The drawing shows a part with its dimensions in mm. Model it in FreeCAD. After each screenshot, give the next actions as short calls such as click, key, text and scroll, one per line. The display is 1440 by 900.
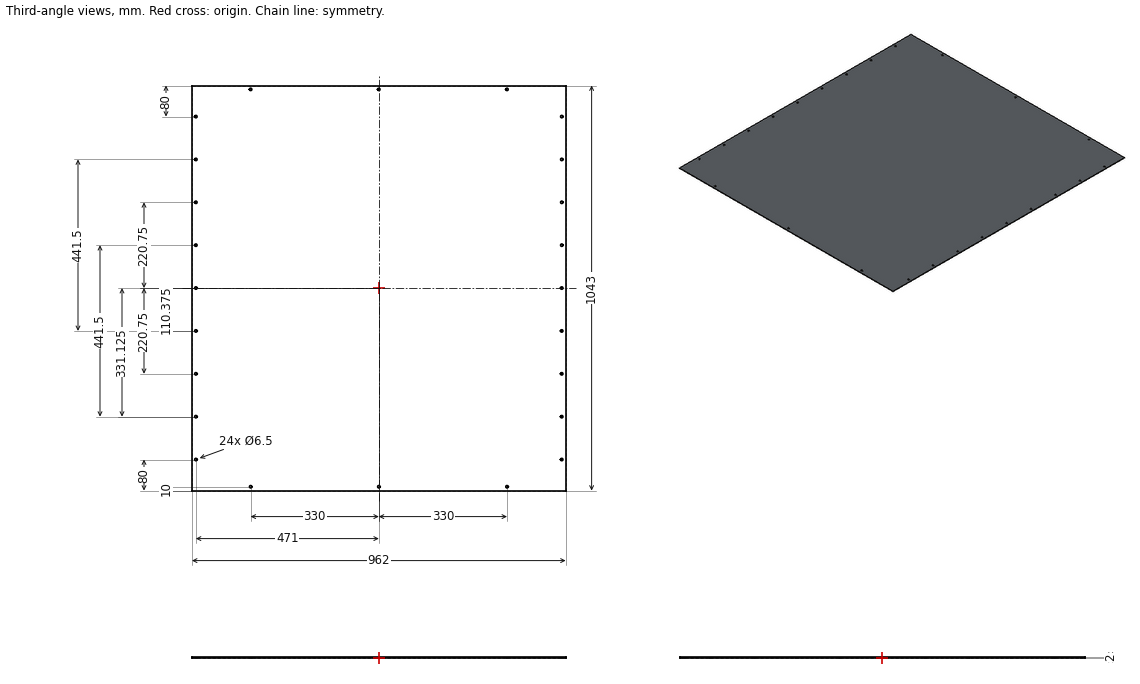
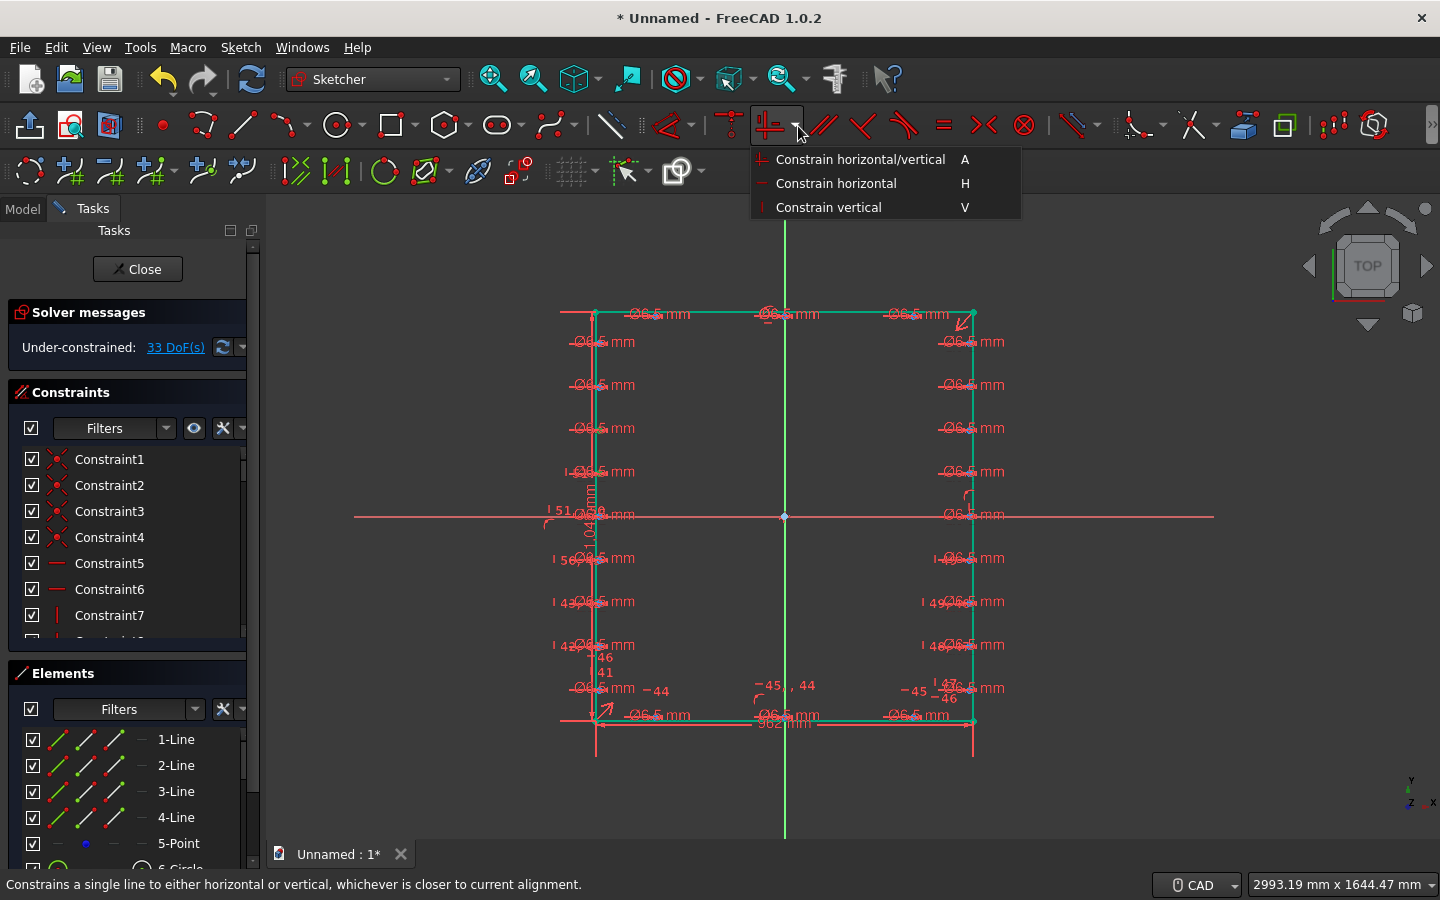
click(886, 207)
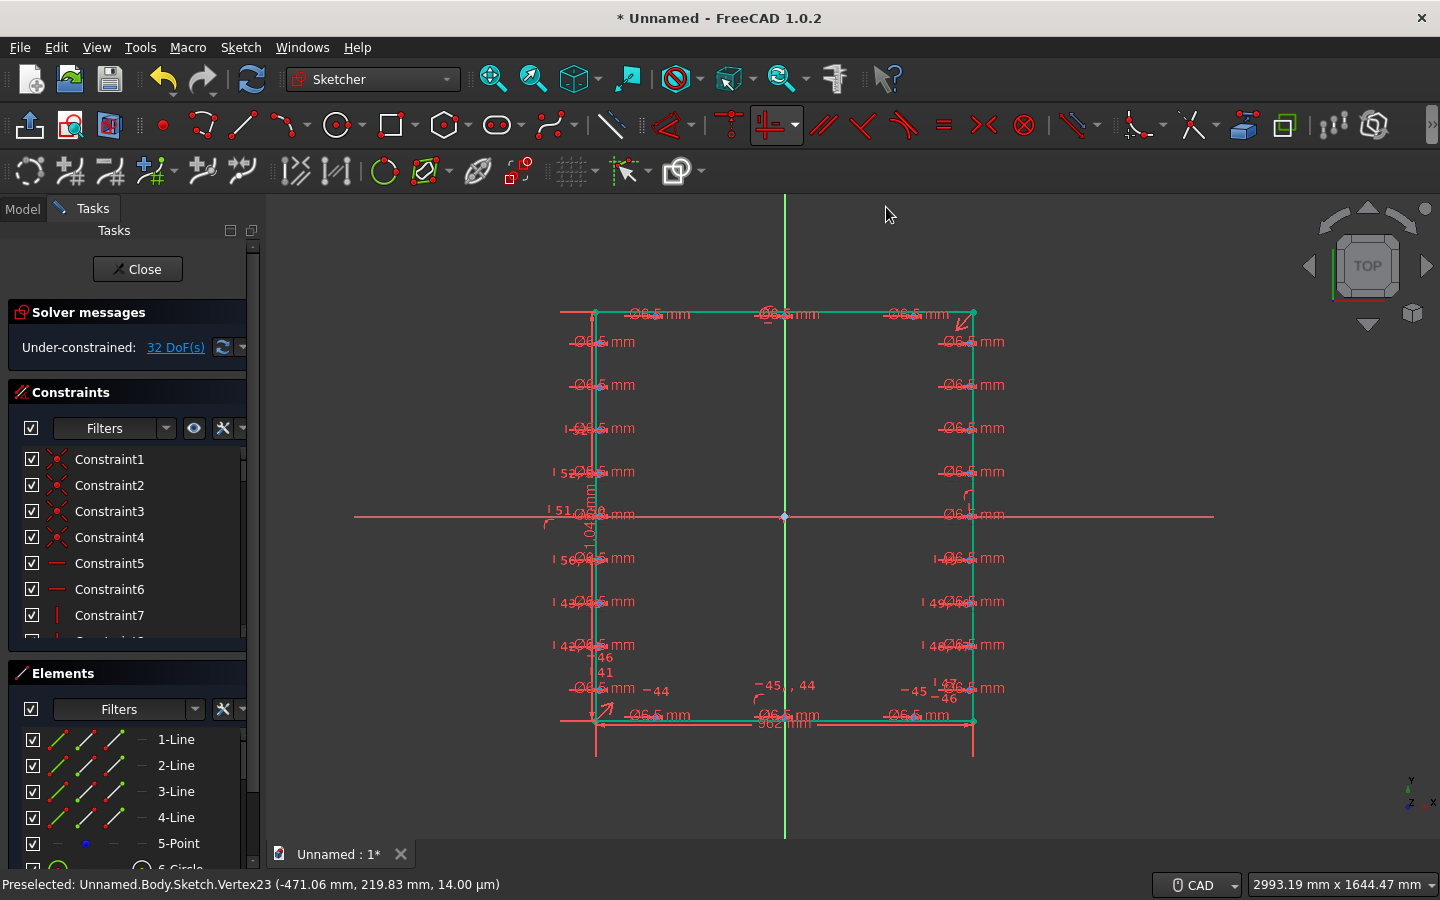
click(600, 430)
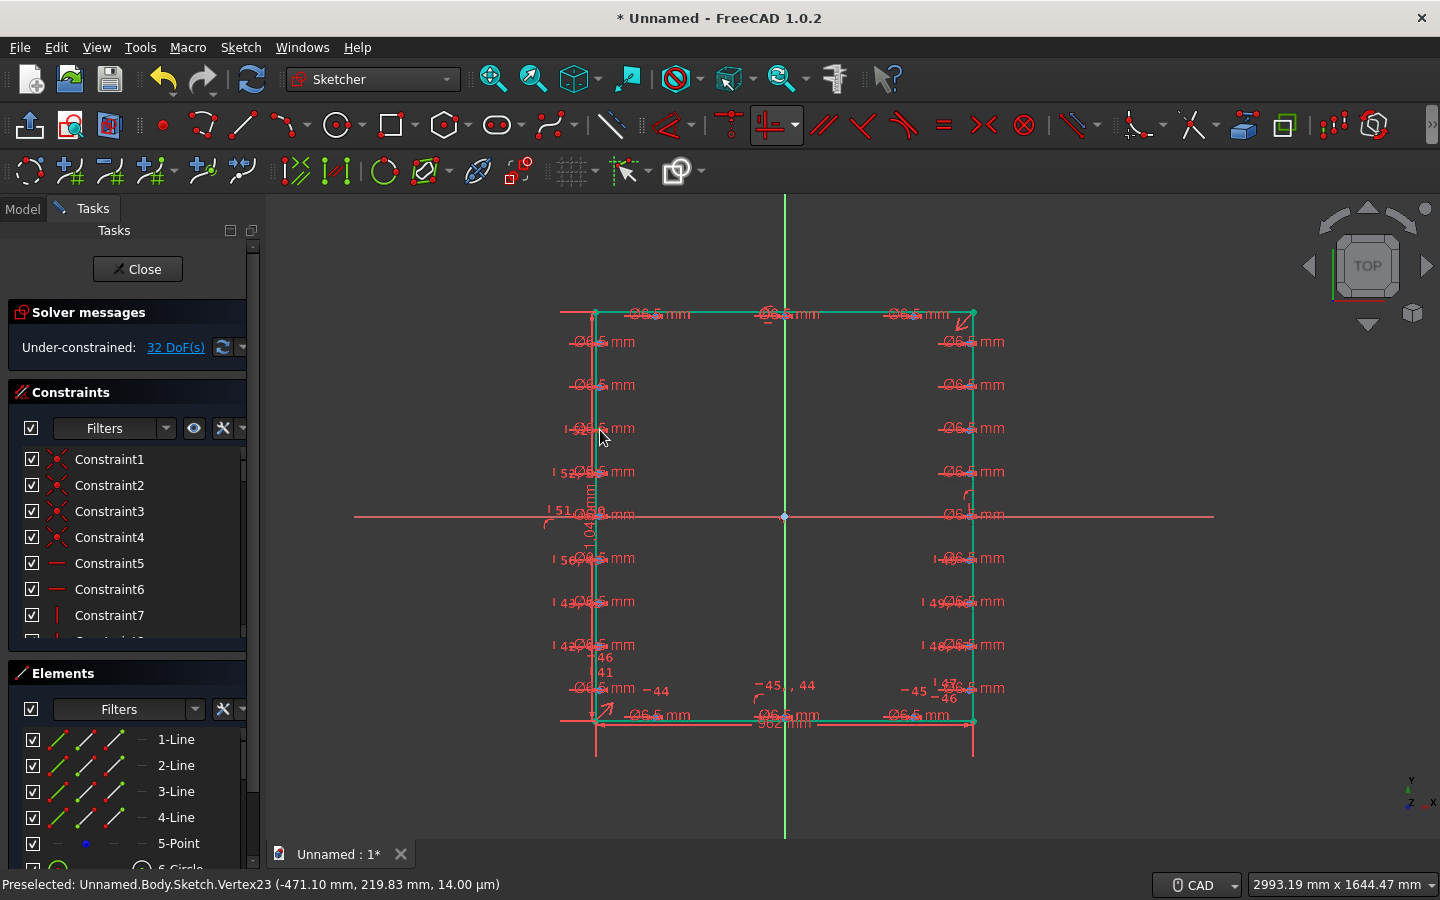
click(600, 387)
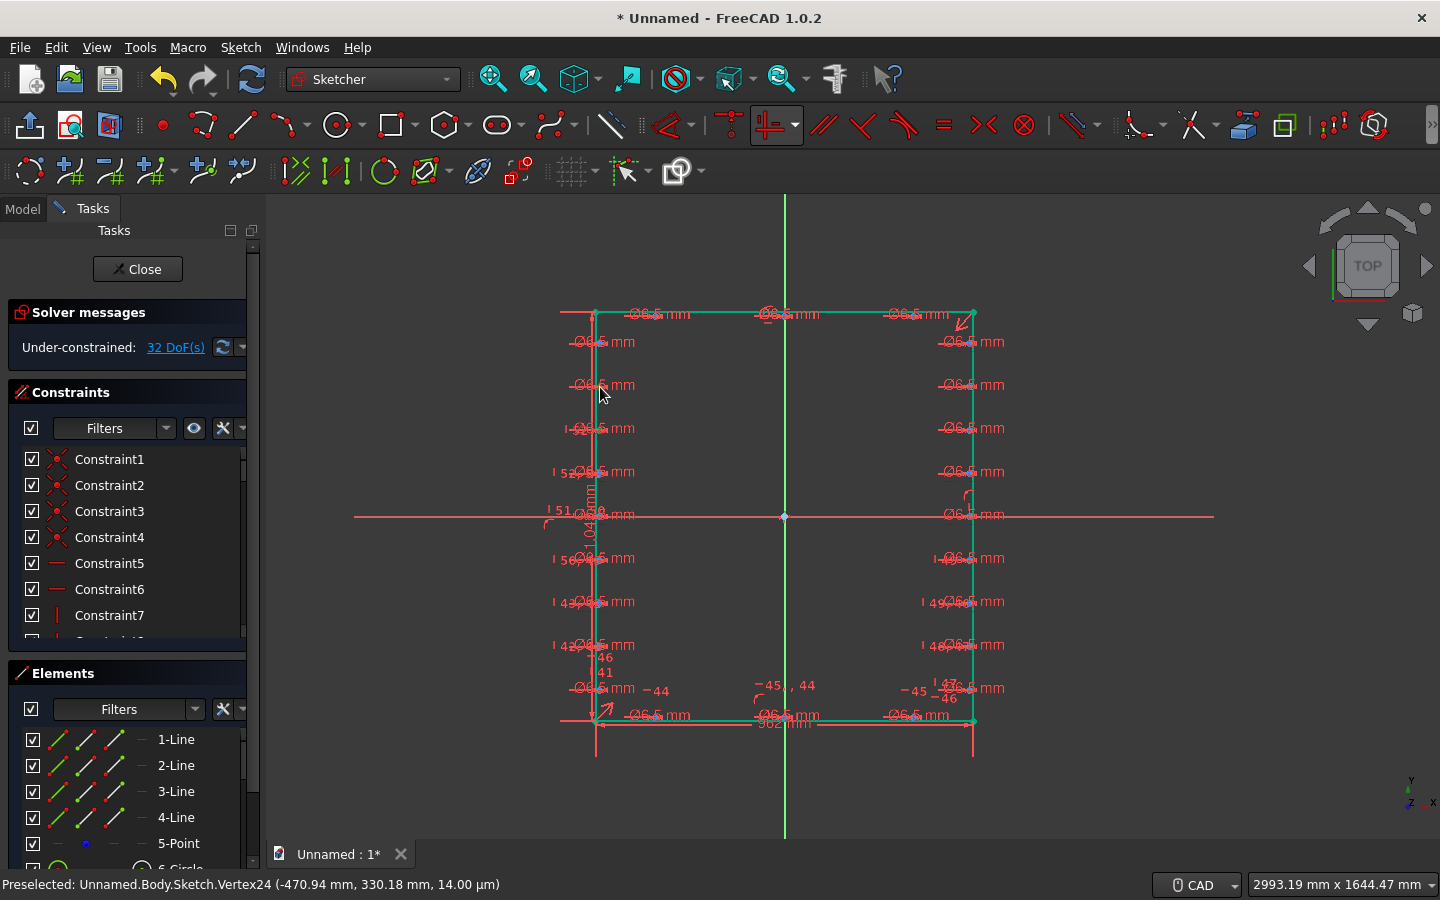
click(798, 126)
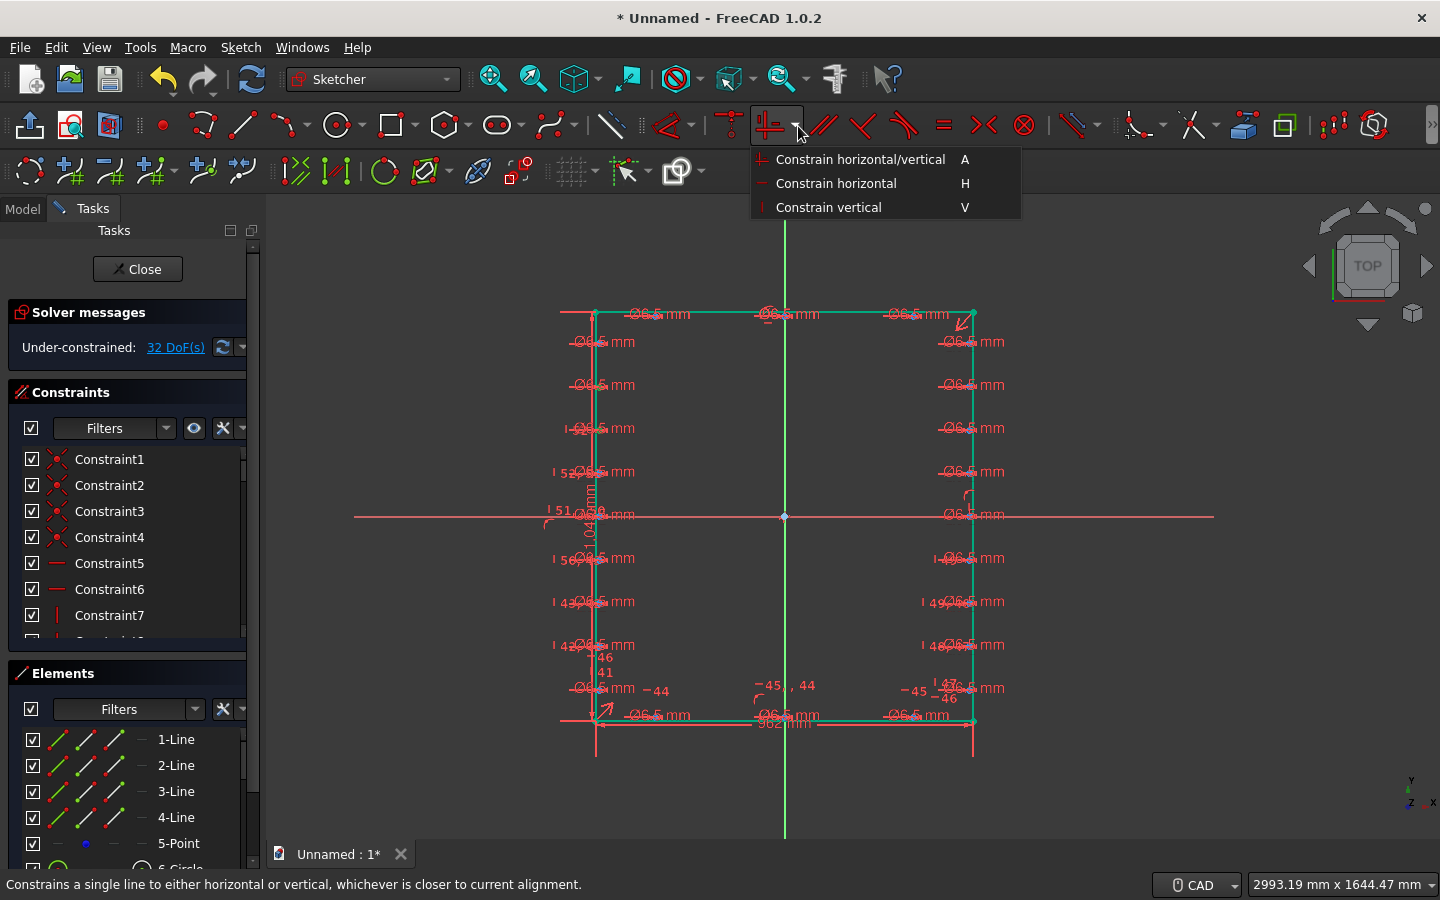
click(886, 207)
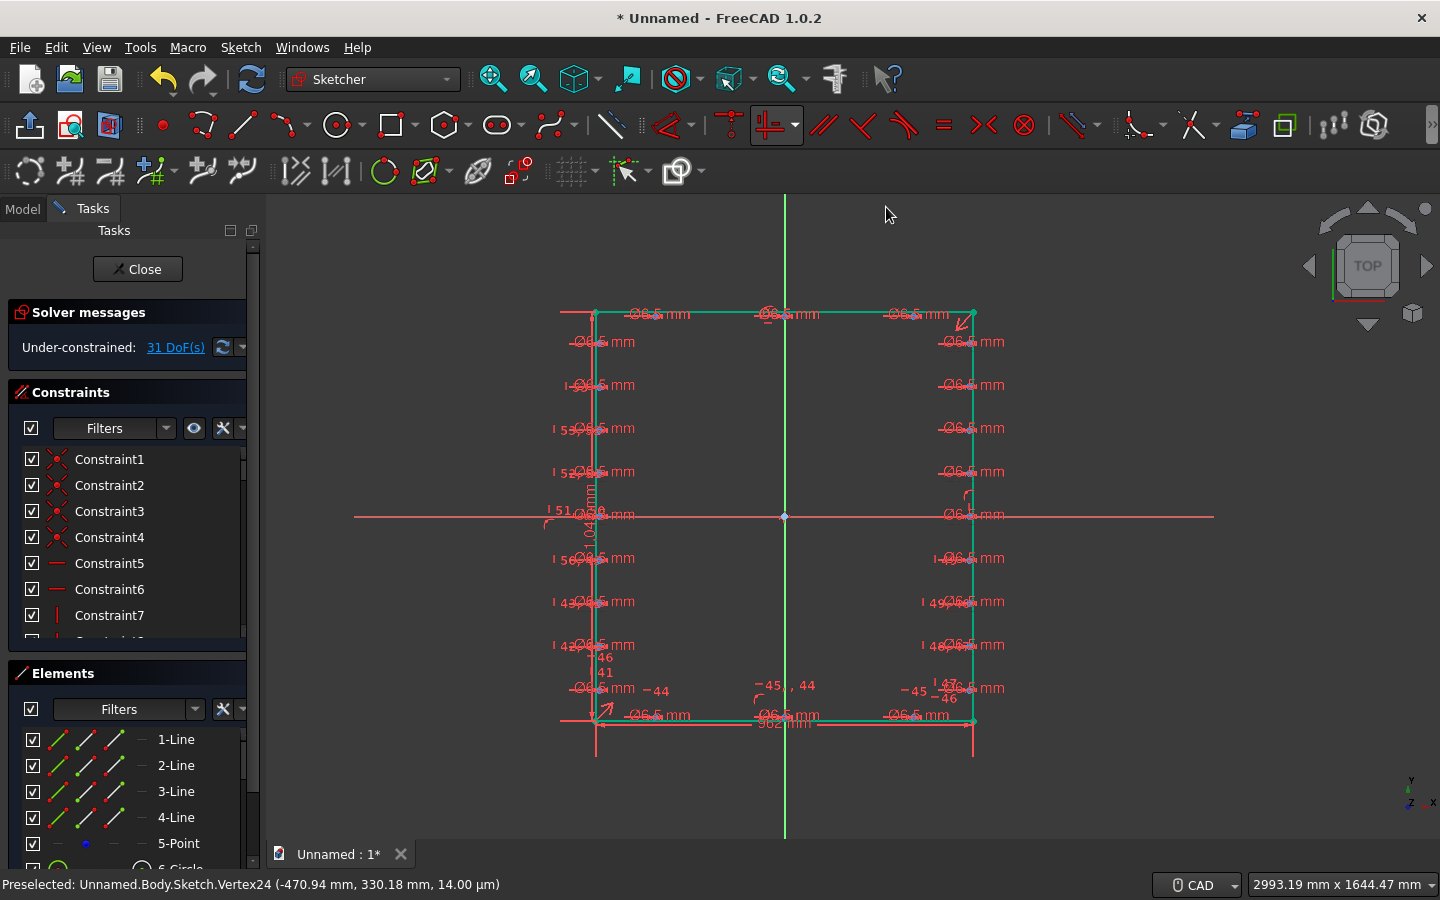
click(600, 387)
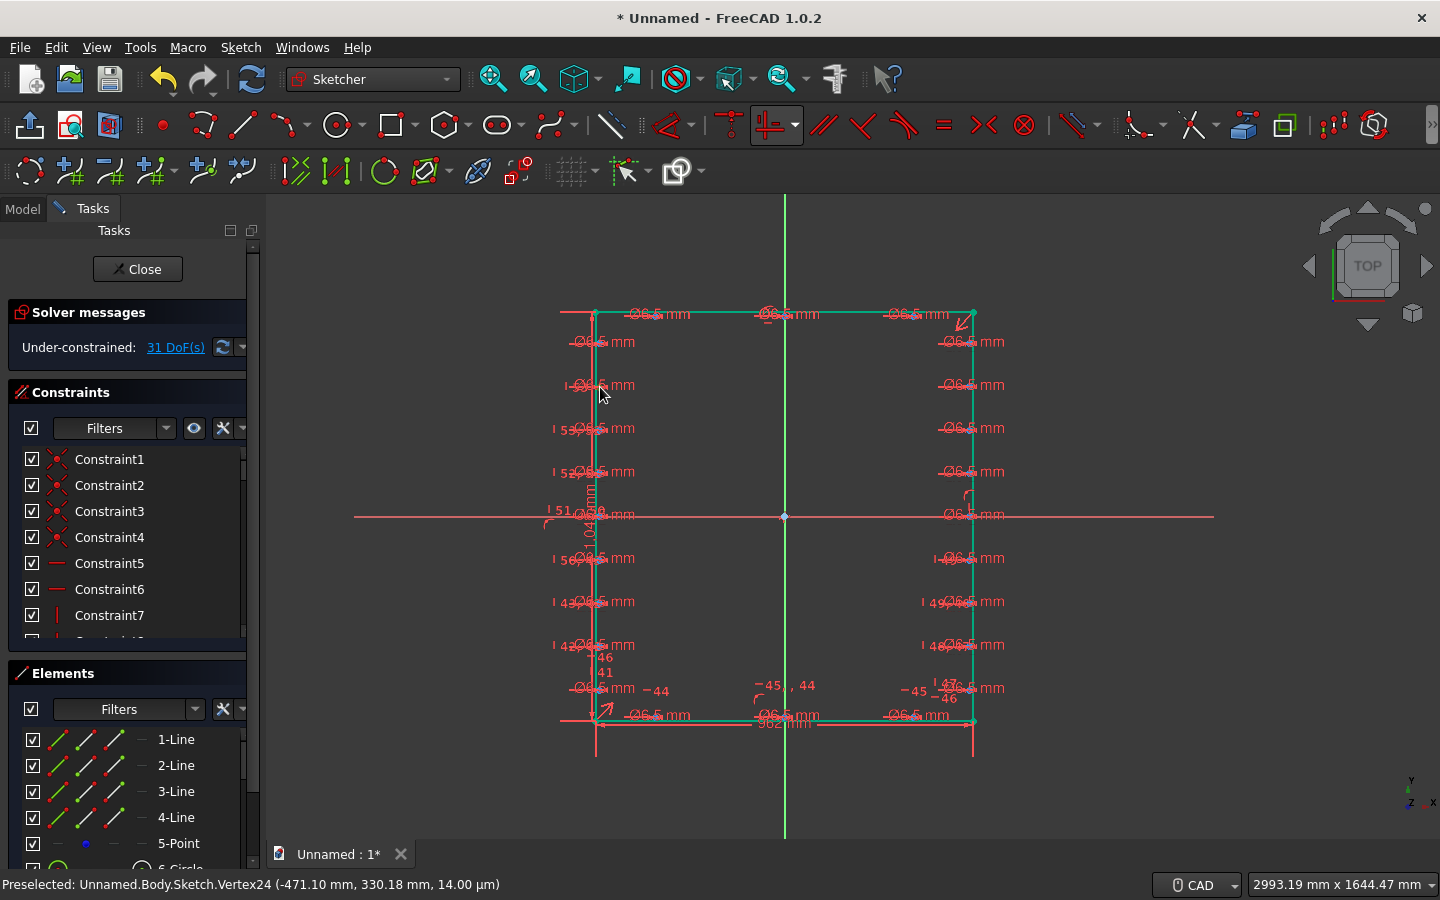
click(600, 344)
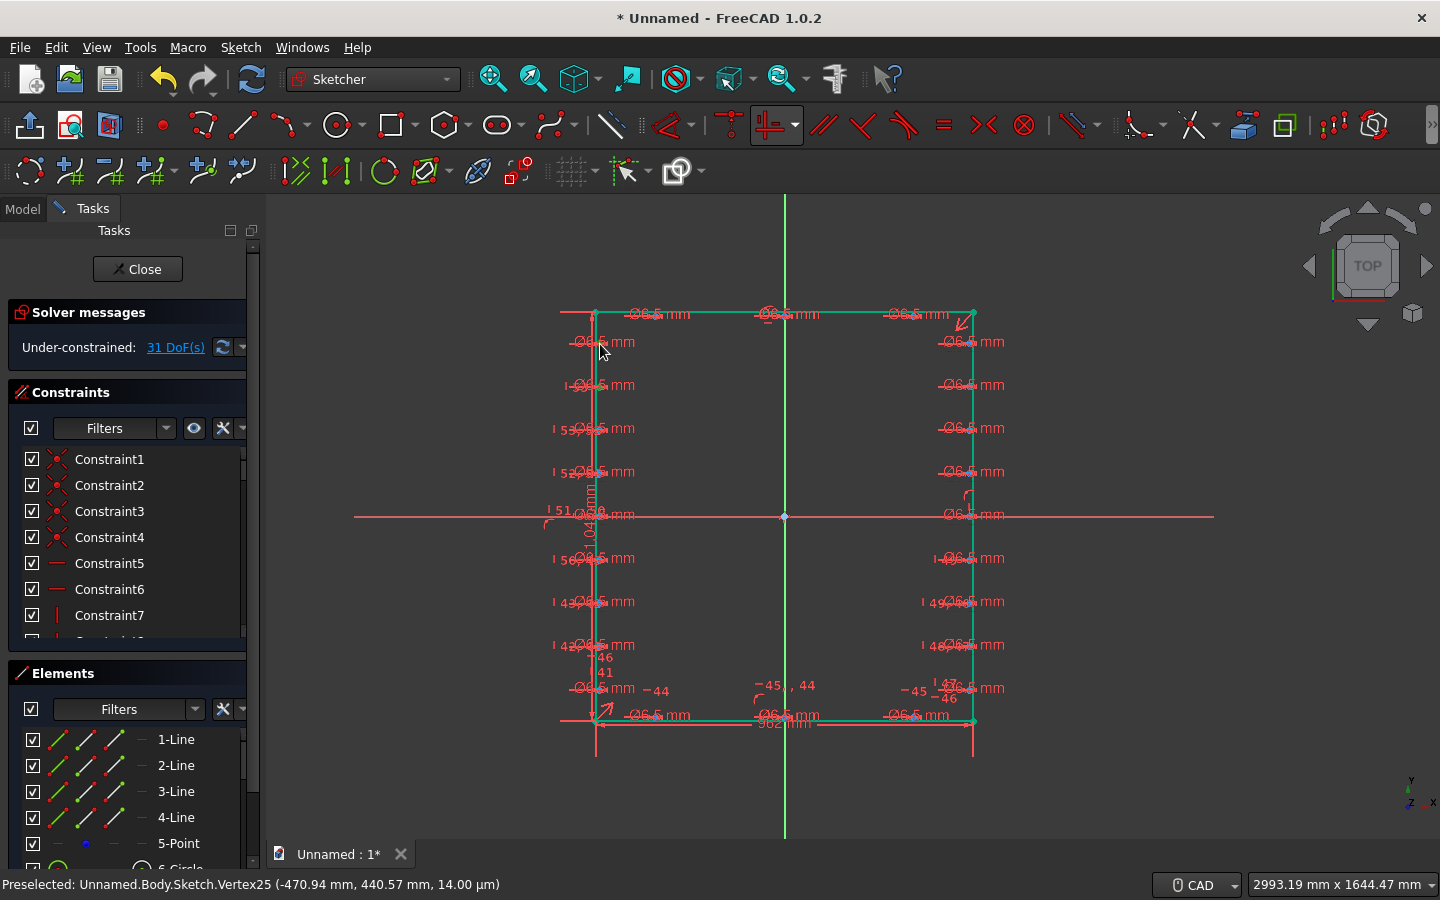
key(v)